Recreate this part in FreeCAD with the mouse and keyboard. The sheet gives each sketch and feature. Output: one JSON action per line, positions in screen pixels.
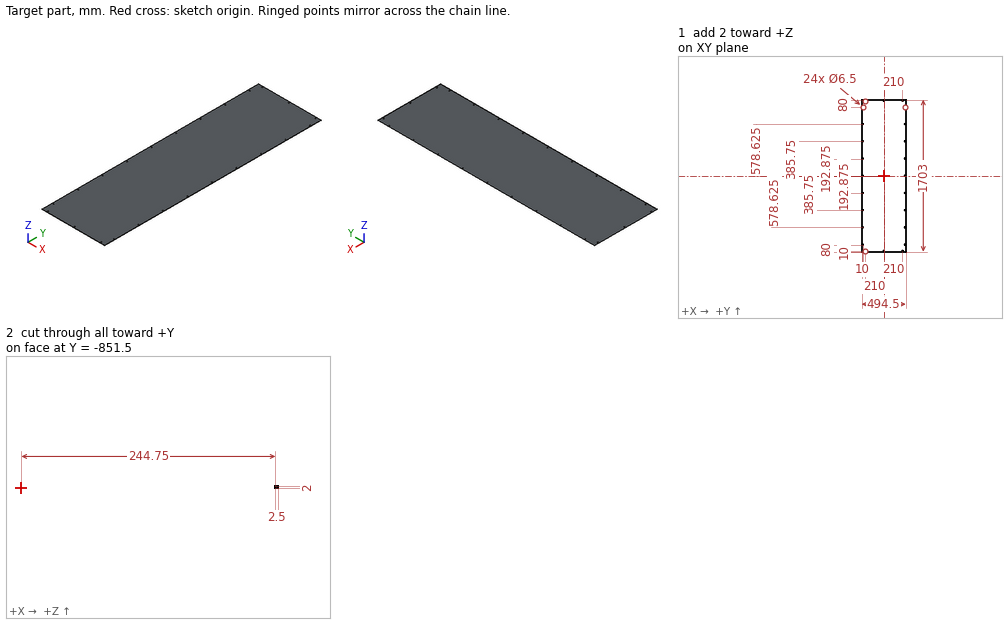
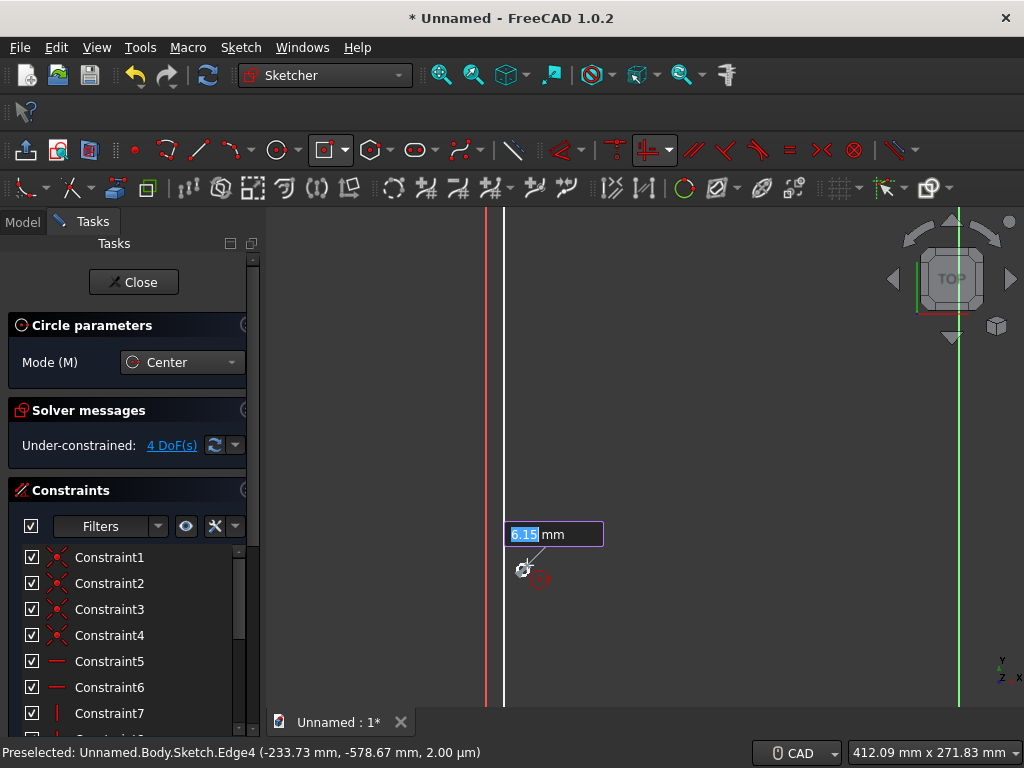
{"action": "type", "text": "6.5"}
{"action": "key", "text": "Return"}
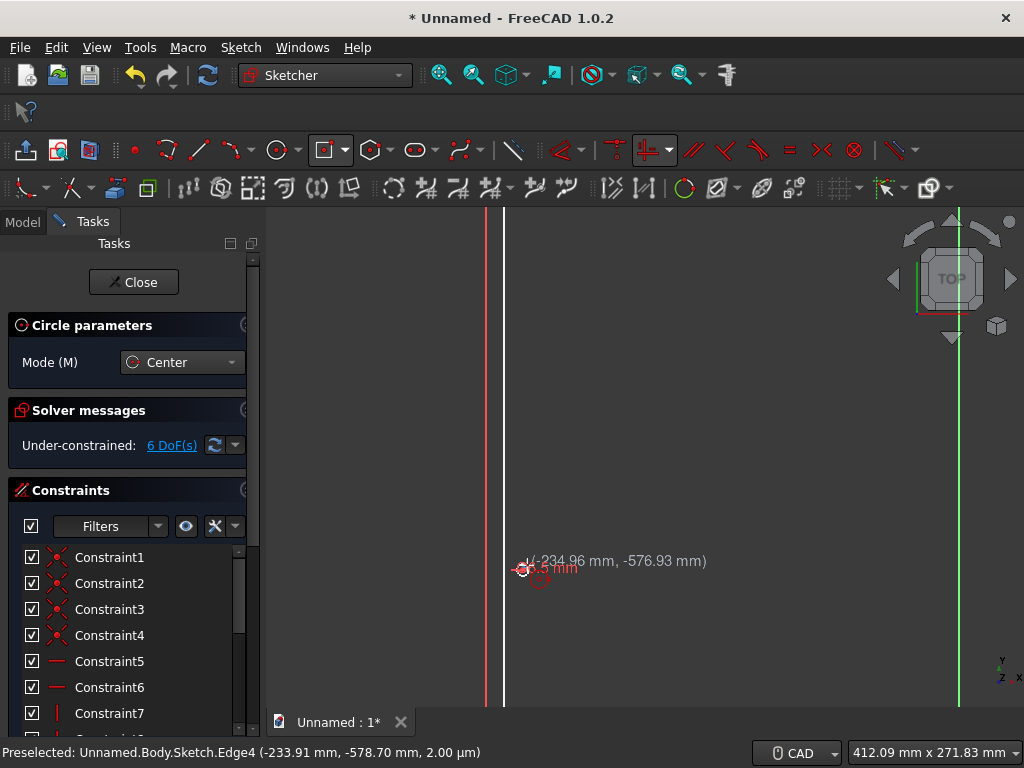
{"action": "scroll", "coordinate": [538, 552], "scroll_direction": "down", "scroll_amount": 12}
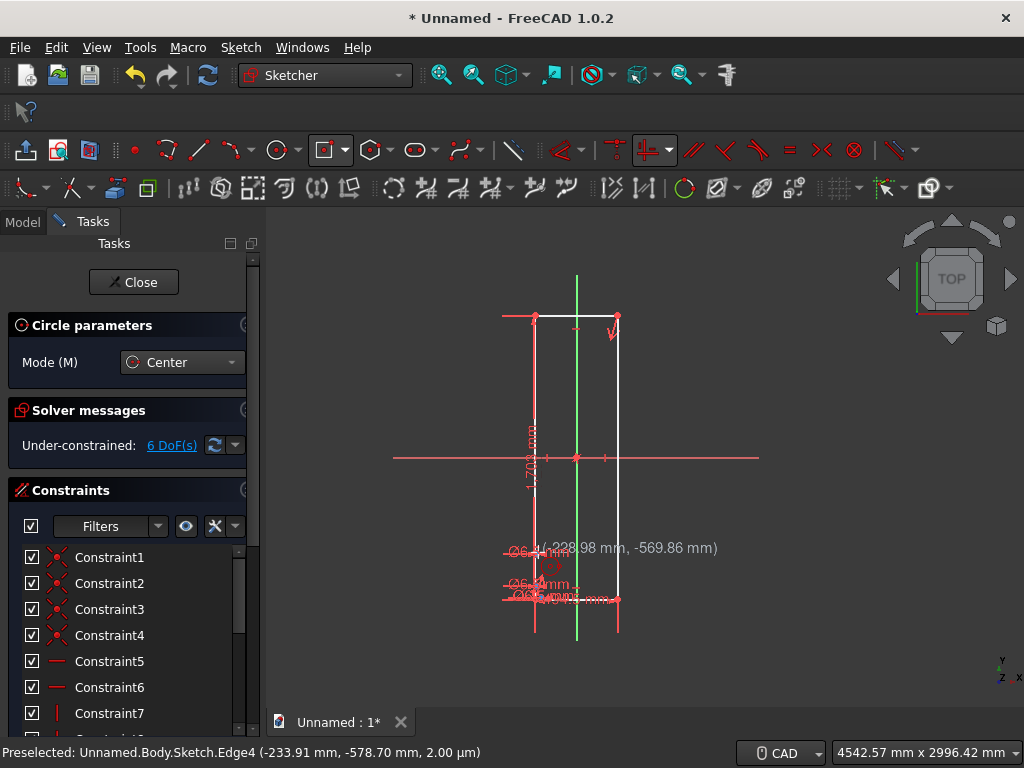
{"action": "scroll", "coordinate": [537, 522], "scroll_direction": "up", "scroll_amount": 19}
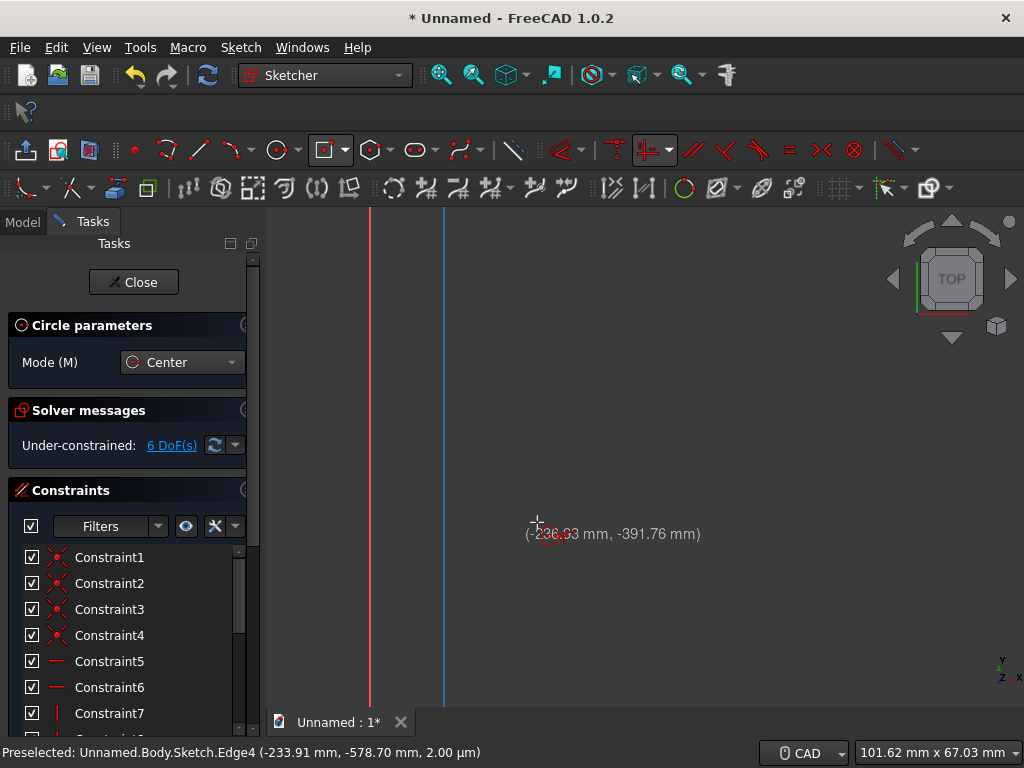
{"action": "scroll", "coordinate": [528, 537], "scroll_direction": "down", "scroll_amount": 18}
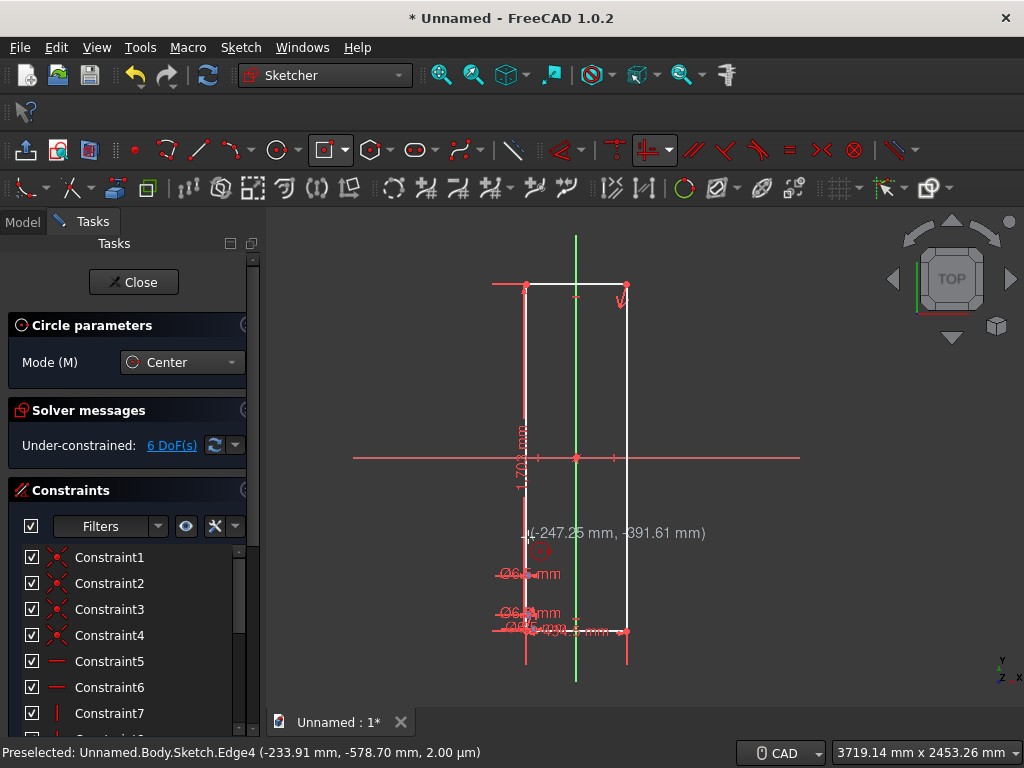
{"action": "scroll", "coordinate": [528, 536], "scroll_direction": "up", "scroll_amount": 11}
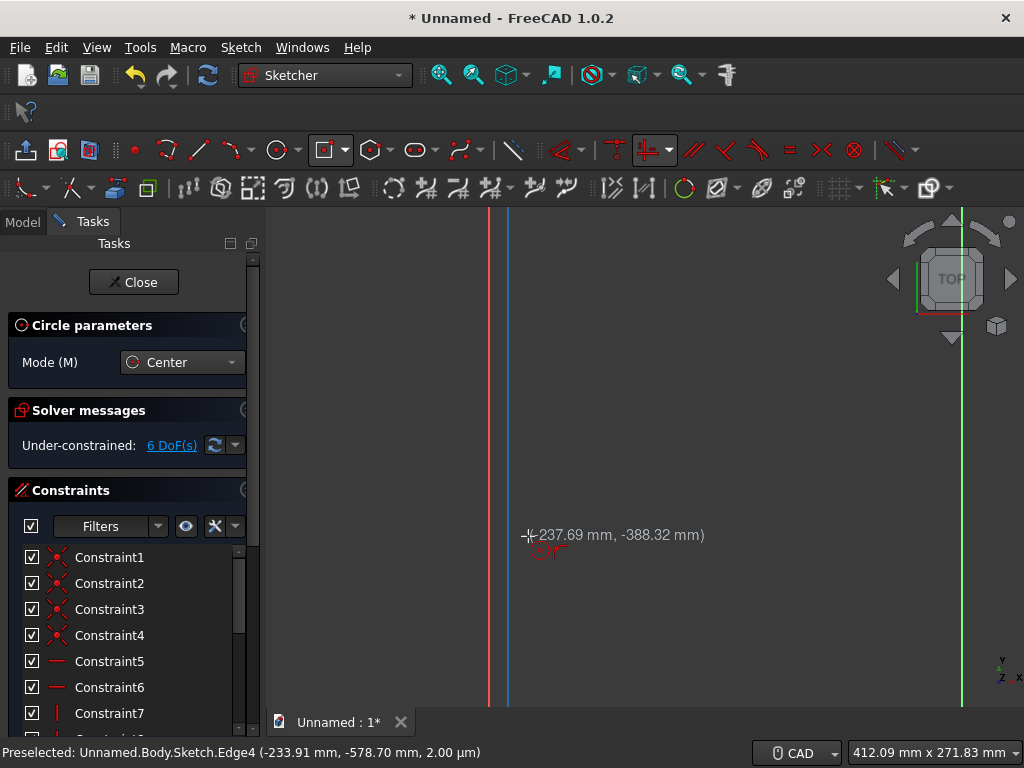
{"action": "left_click", "coordinate": [526, 535]}
{"action": "mouse_move", "coordinate": [530, 531]}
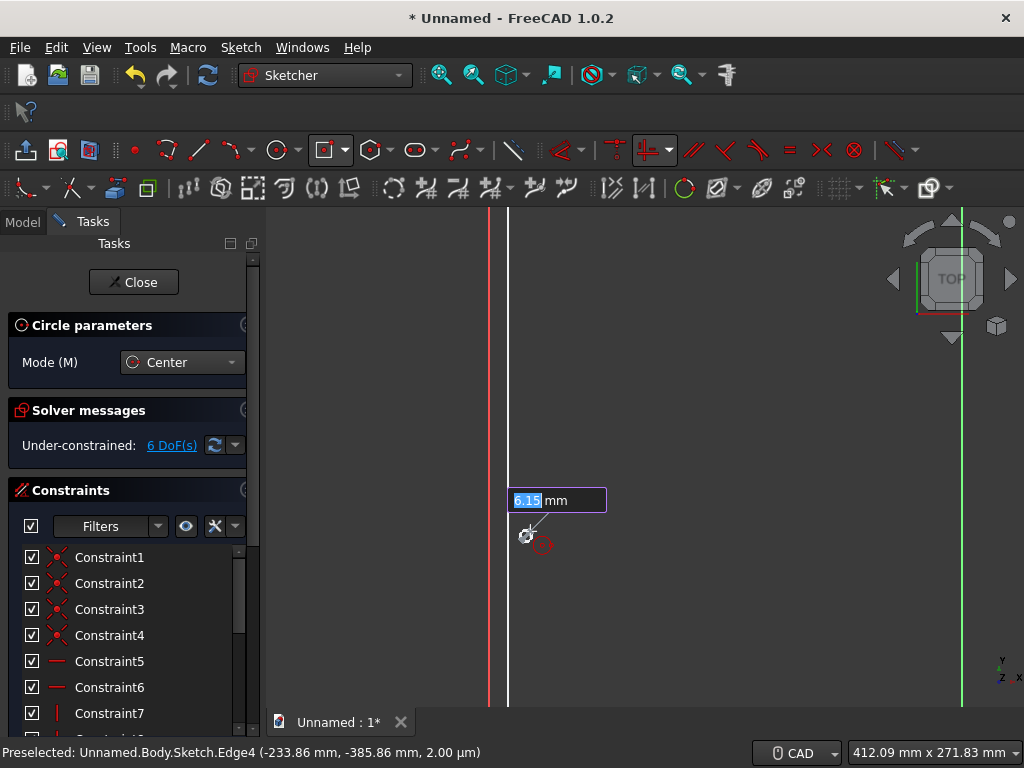
{"action": "type", "text": "6.5"}
{"action": "key", "text": "Return"}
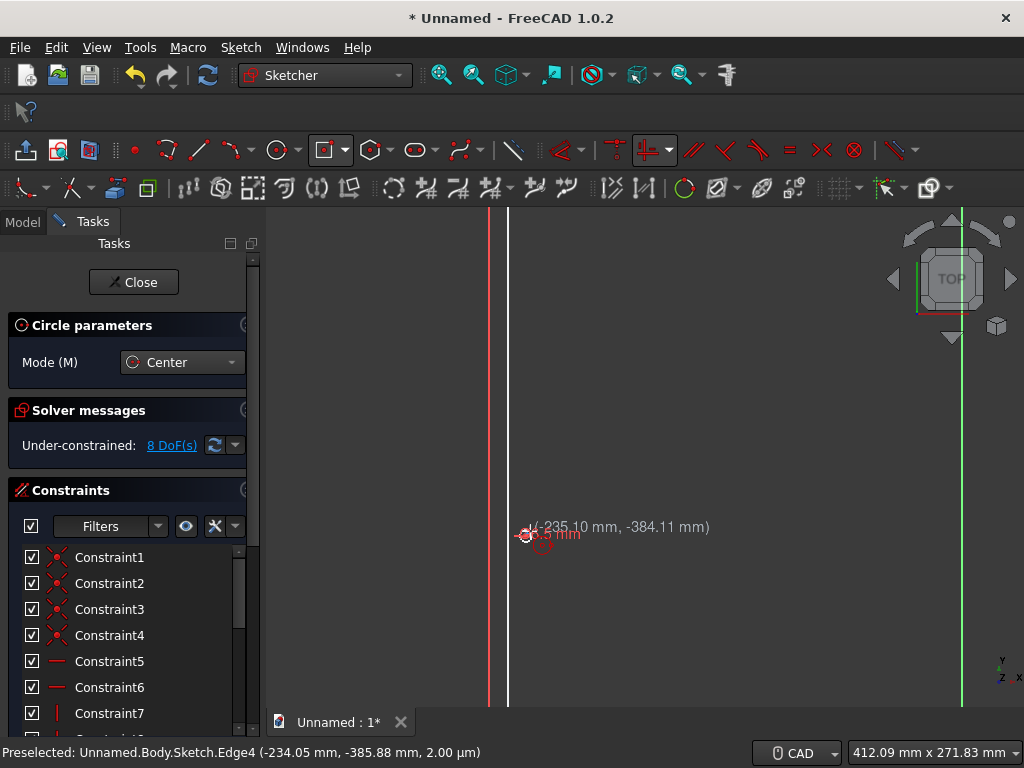
{"action": "scroll", "coordinate": [538, 520], "scroll_direction": "down", "scroll_amount": 12}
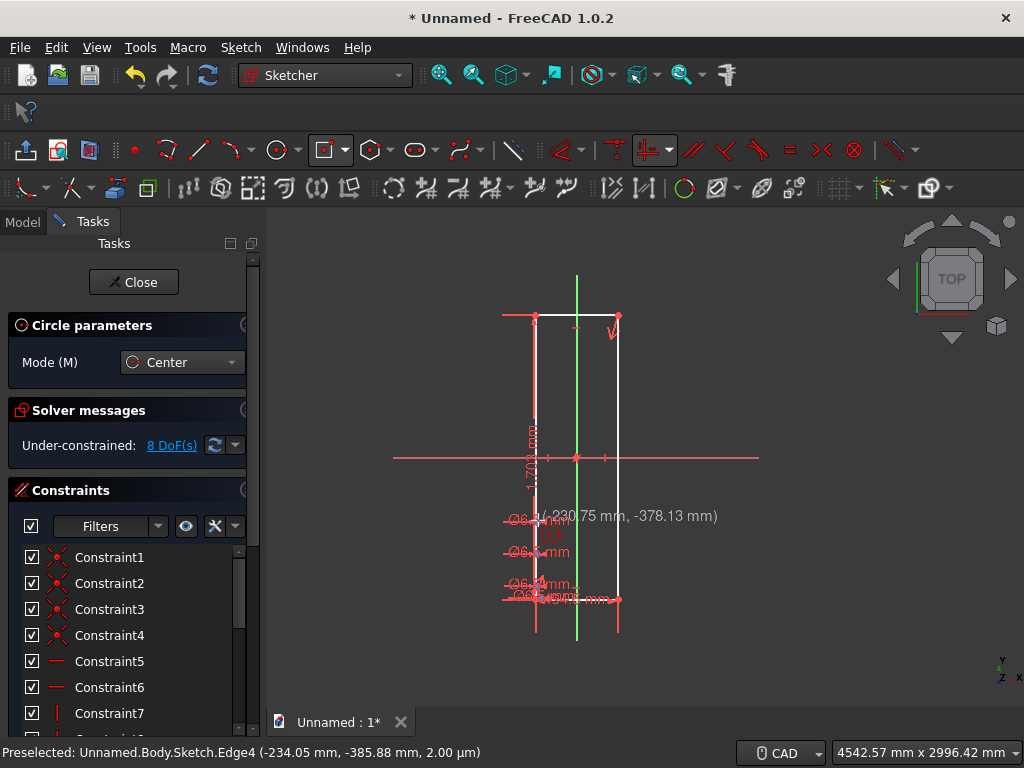
{"action": "scroll", "coordinate": [537, 490], "scroll_direction": "up", "scroll_amount": 19}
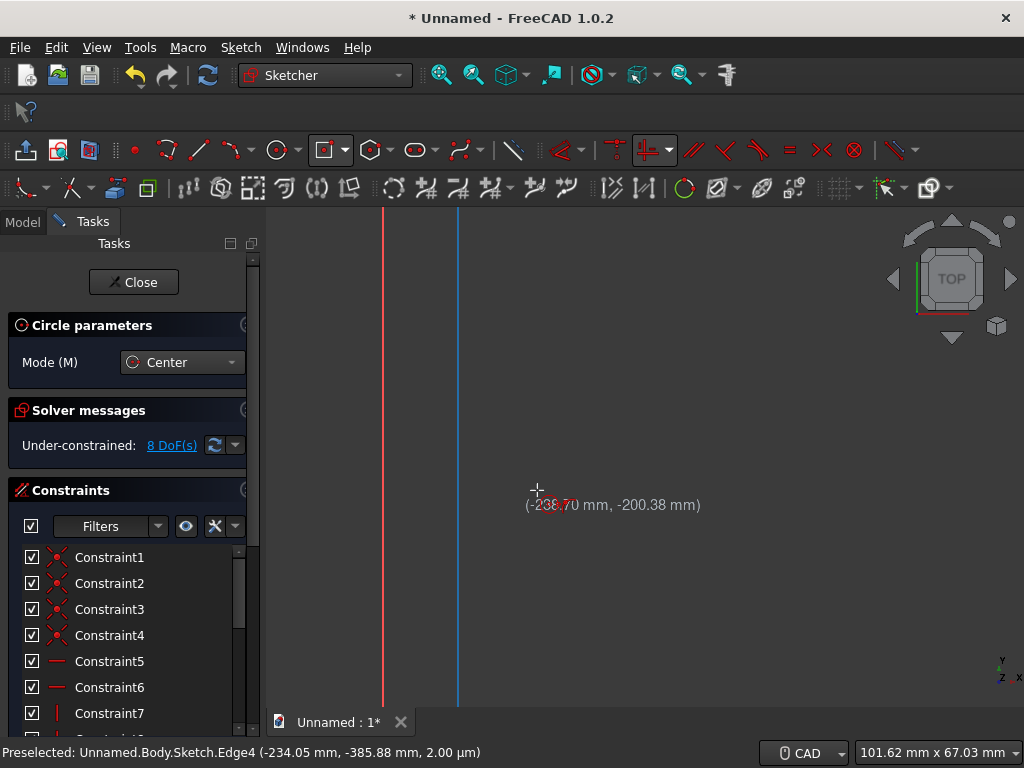
{"action": "scroll", "coordinate": [528, 498], "scroll_direction": "down", "scroll_amount": 18}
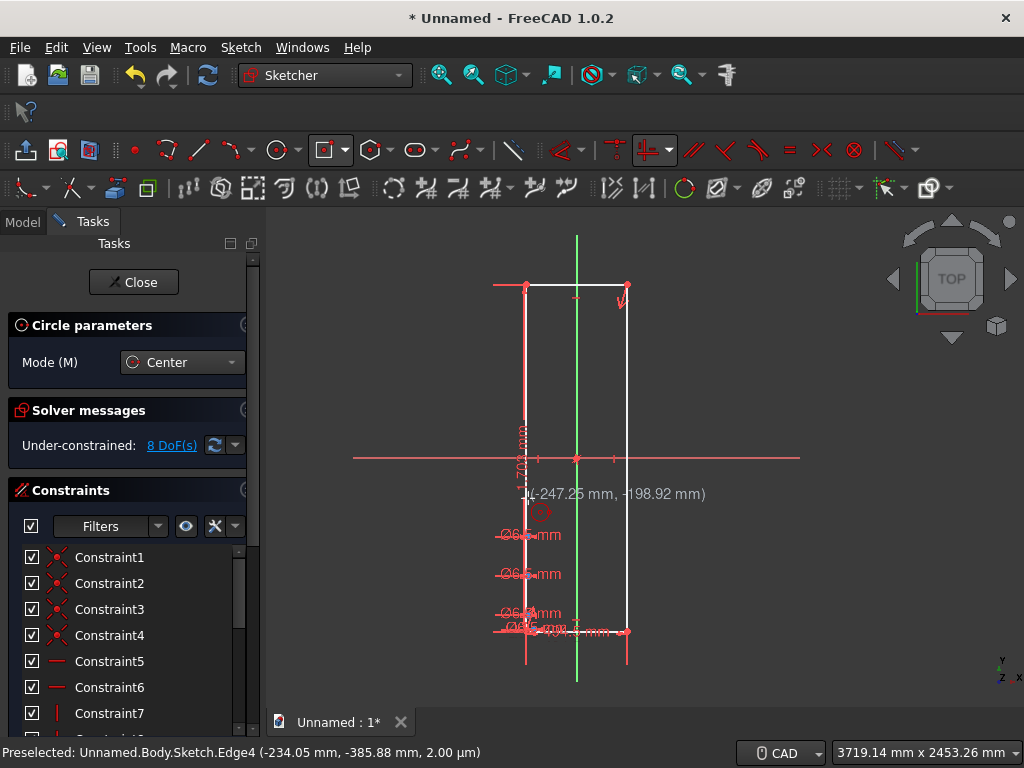
{"action": "scroll", "coordinate": [528, 497], "scroll_direction": "up", "scroll_amount": 11}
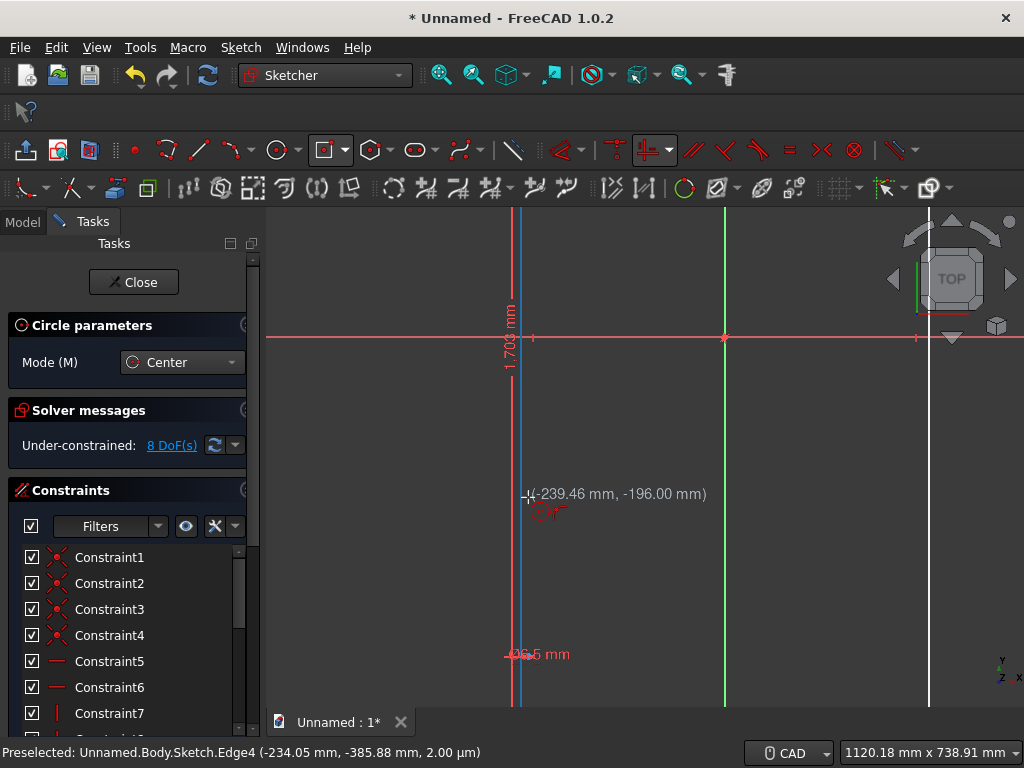
{"action": "left_click", "coordinate": [529, 496]}
{"action": "mouse_move", "coordinate": [534, 491]}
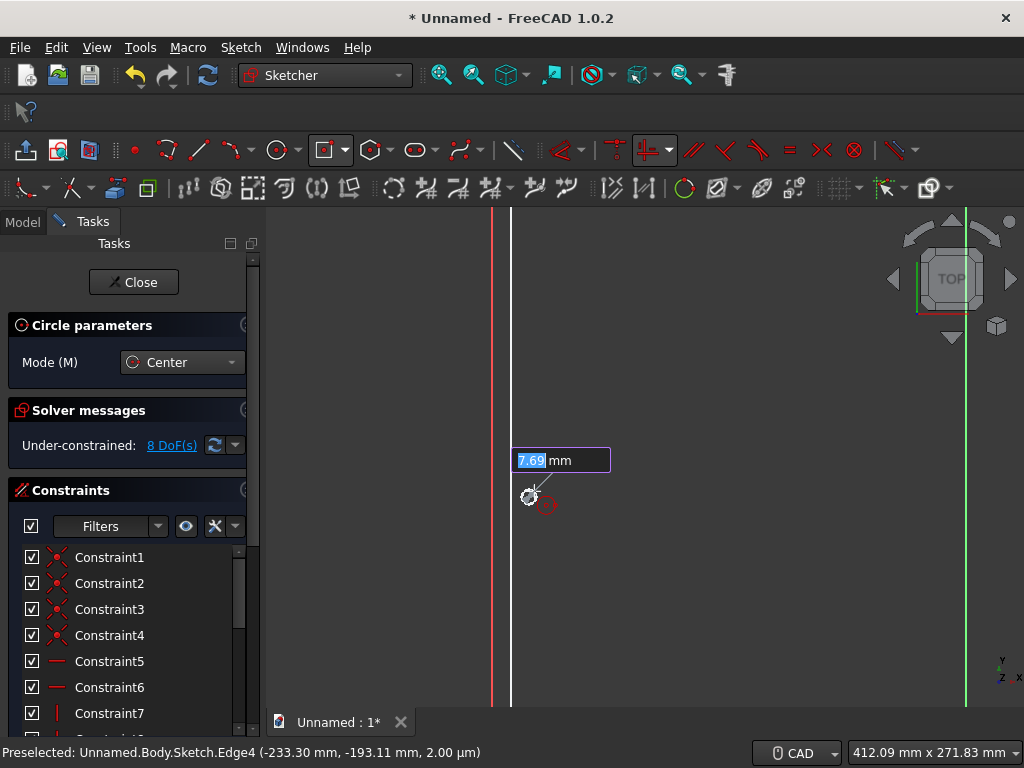
{"action": "type", "text": "6.5"}
{"action": "key", "text": "Return"}